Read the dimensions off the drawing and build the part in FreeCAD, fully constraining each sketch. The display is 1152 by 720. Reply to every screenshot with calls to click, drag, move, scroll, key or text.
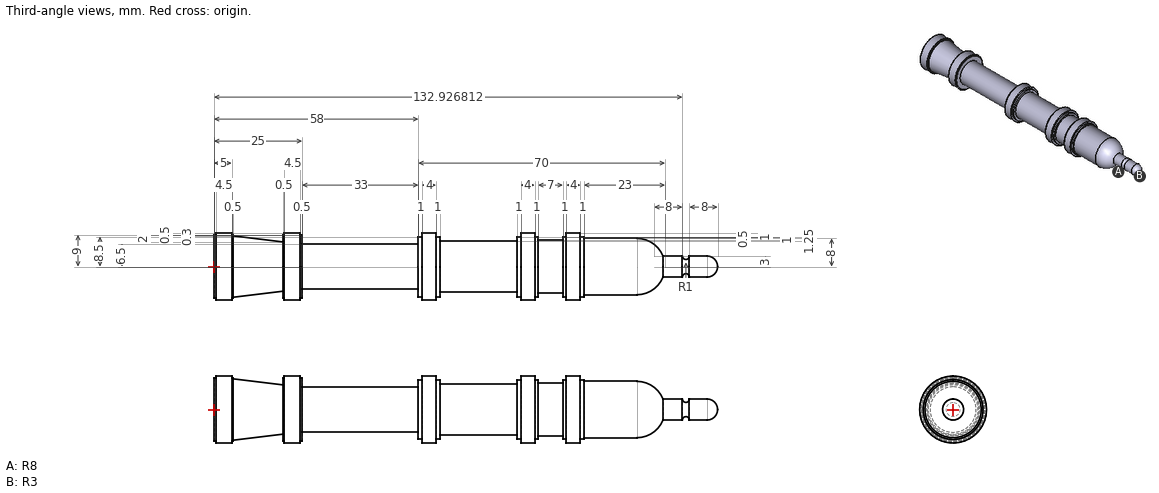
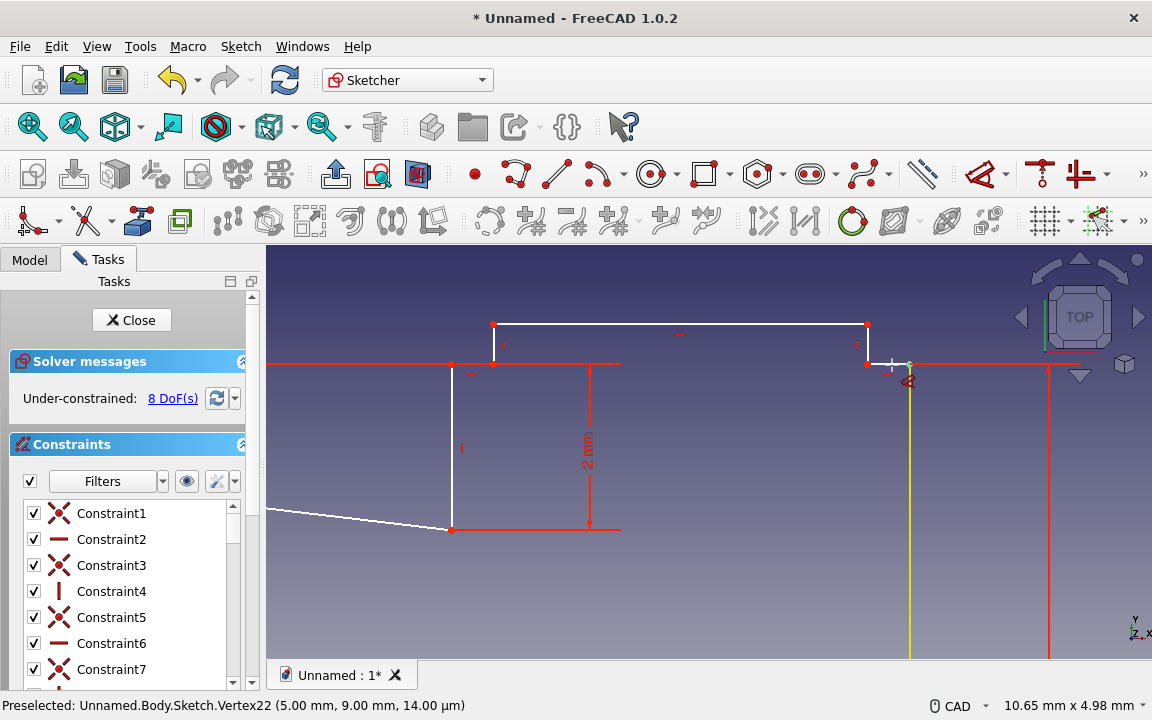
click(889, 364)
click(889, 330)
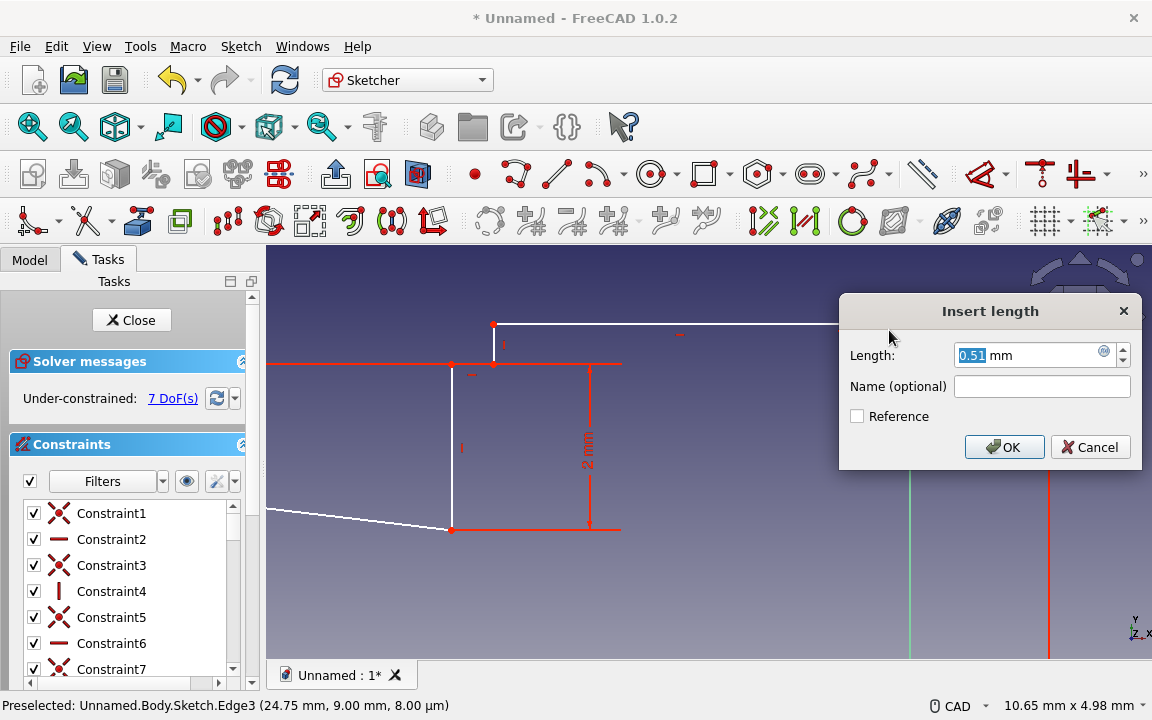
text(0.5)
key(Return)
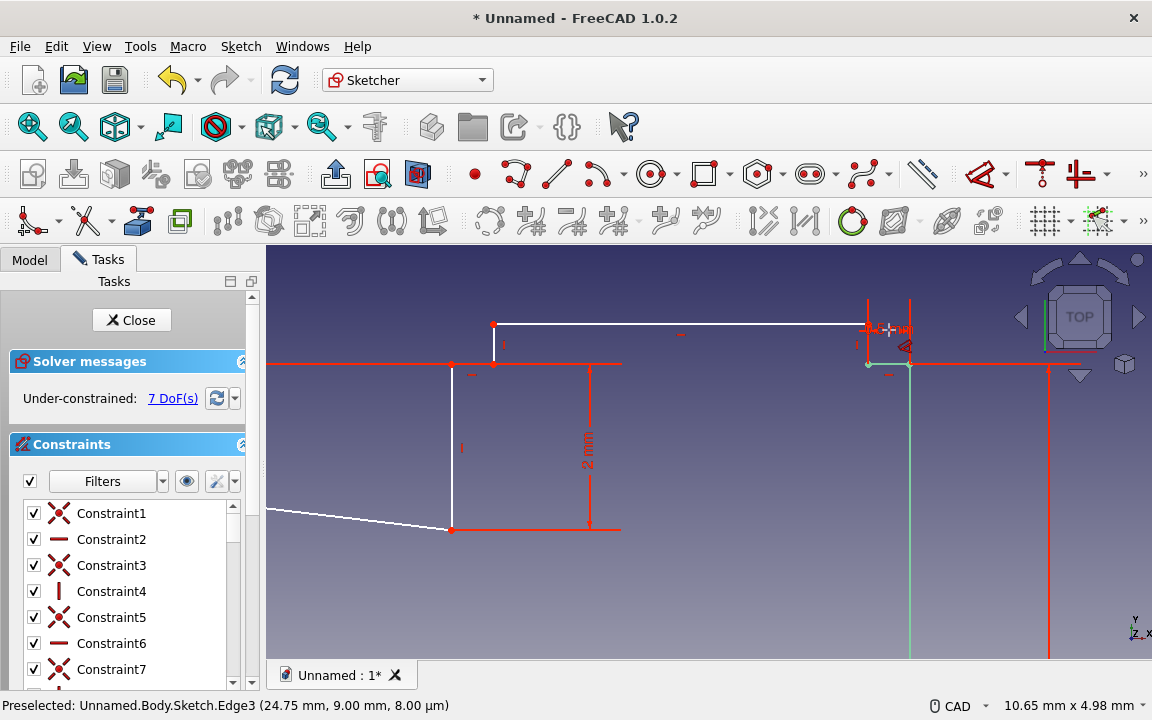
click(868, 352)
click(834, 353)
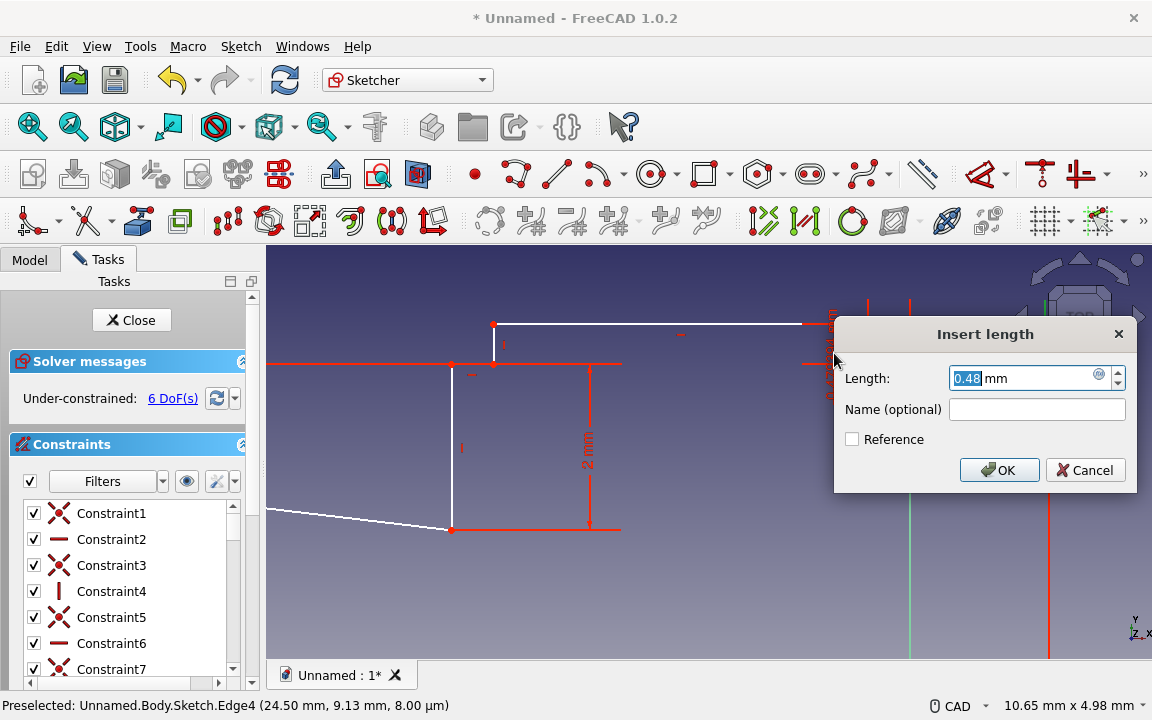
text(0.5)
key(Return)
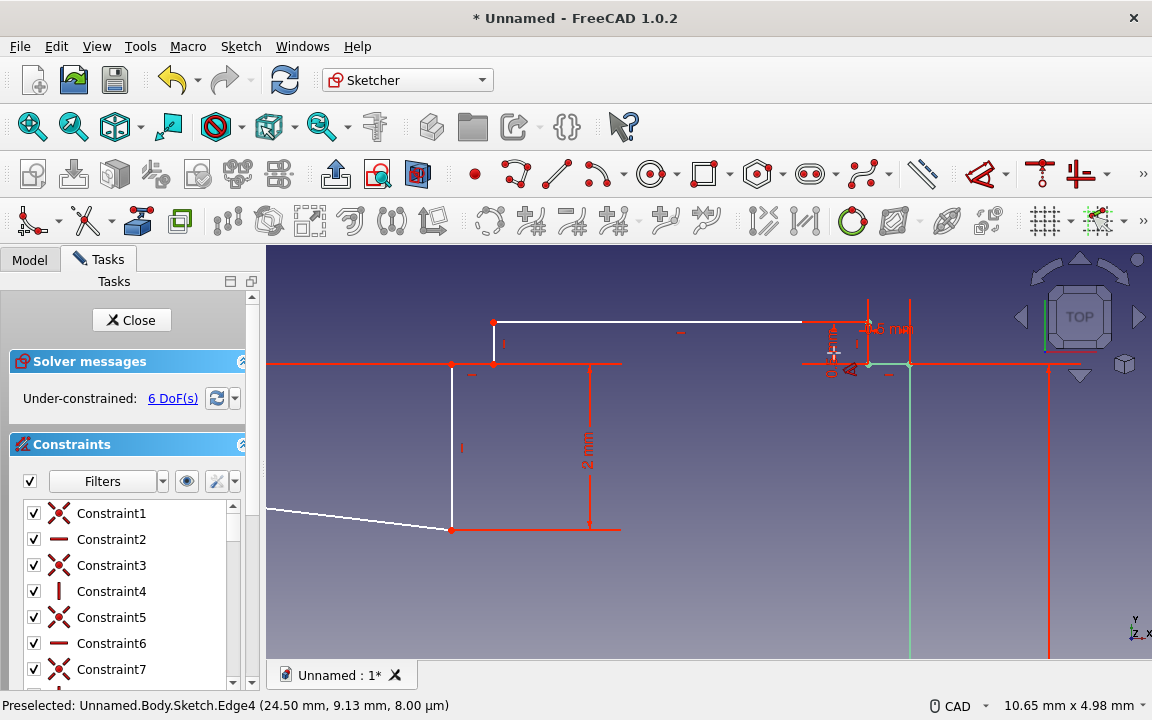
scroll(893, 365, down, 7)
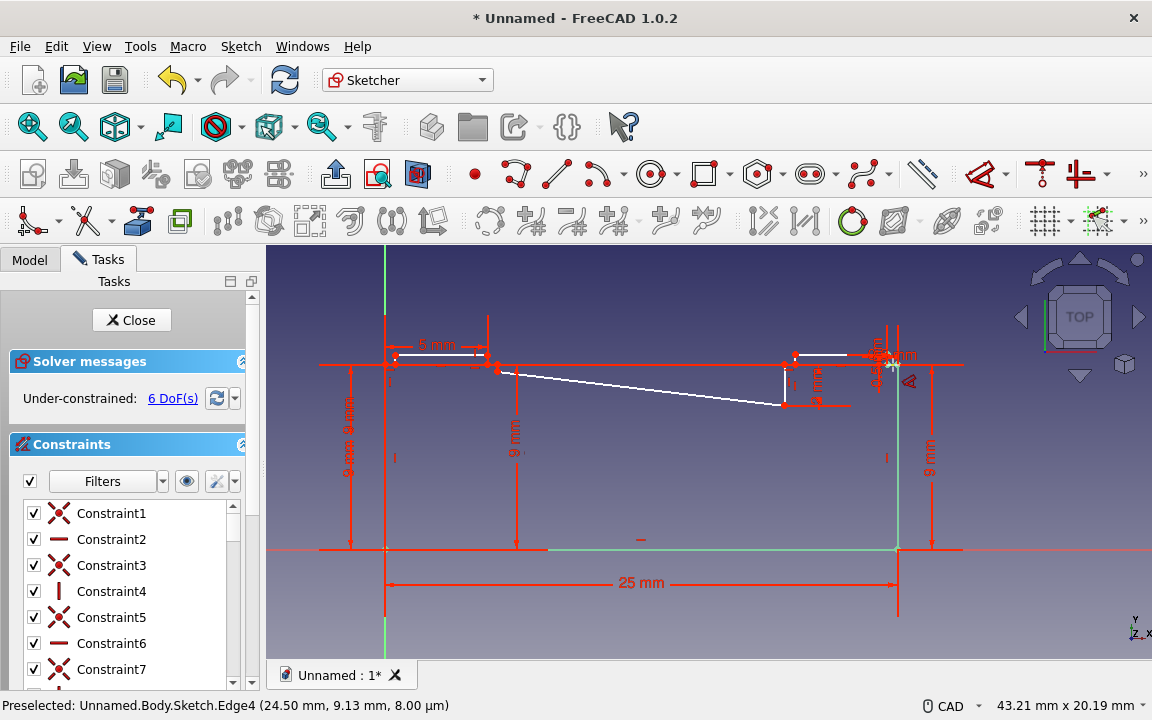
click(860, 355)
click(841, 321)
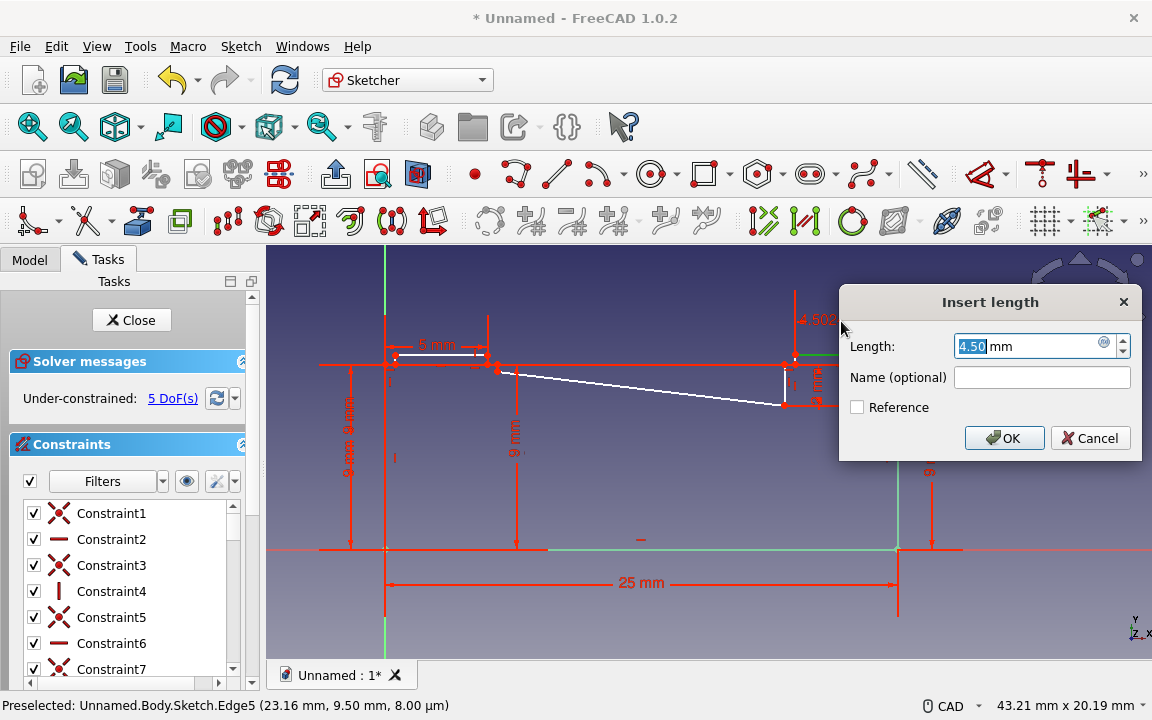
text(4.5)
key(Return)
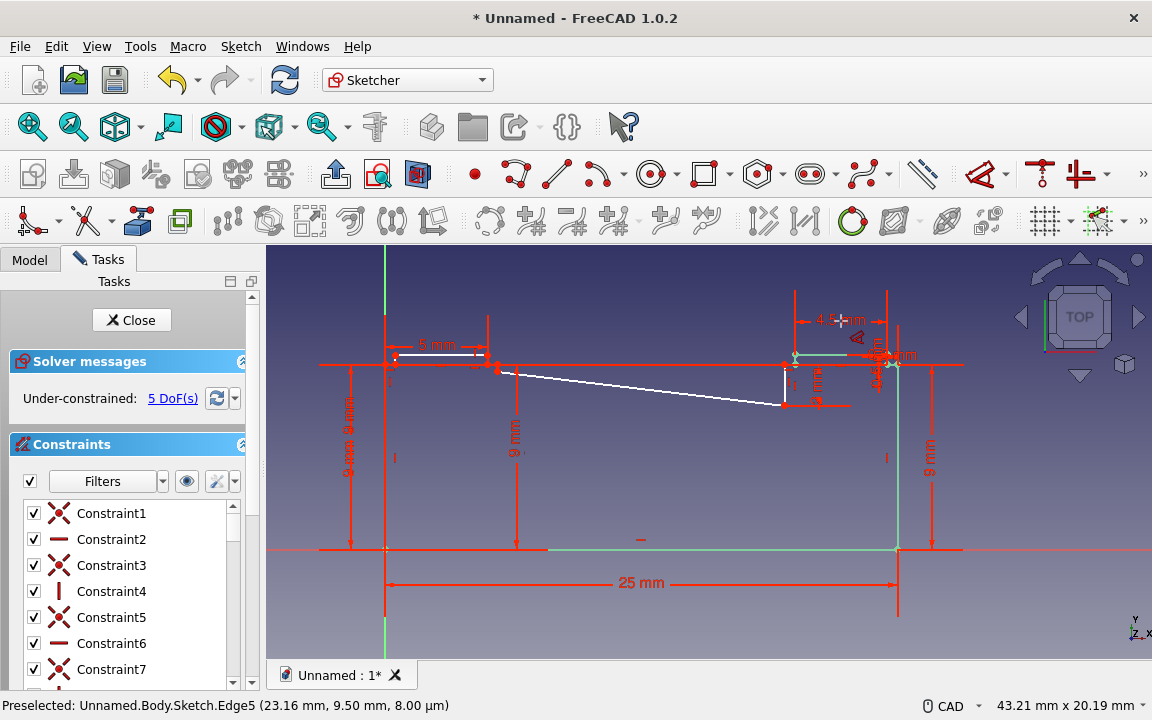
scroll(790, 365, up, 7)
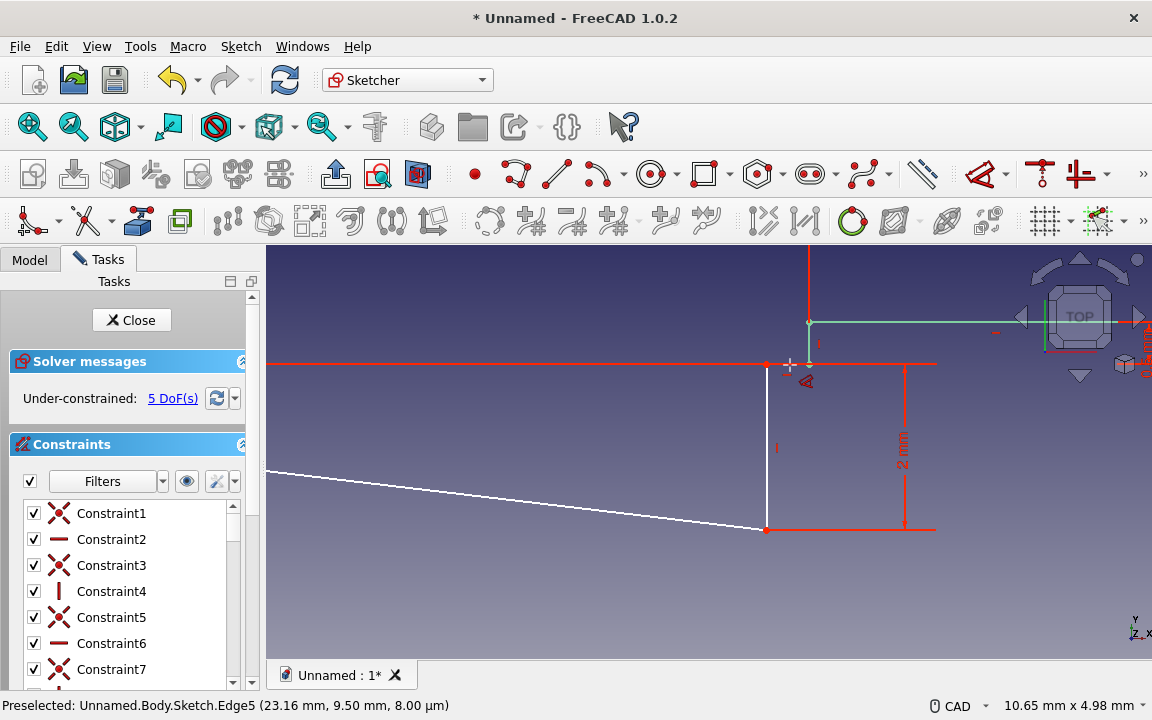
click(788, 364)
click(788, 330)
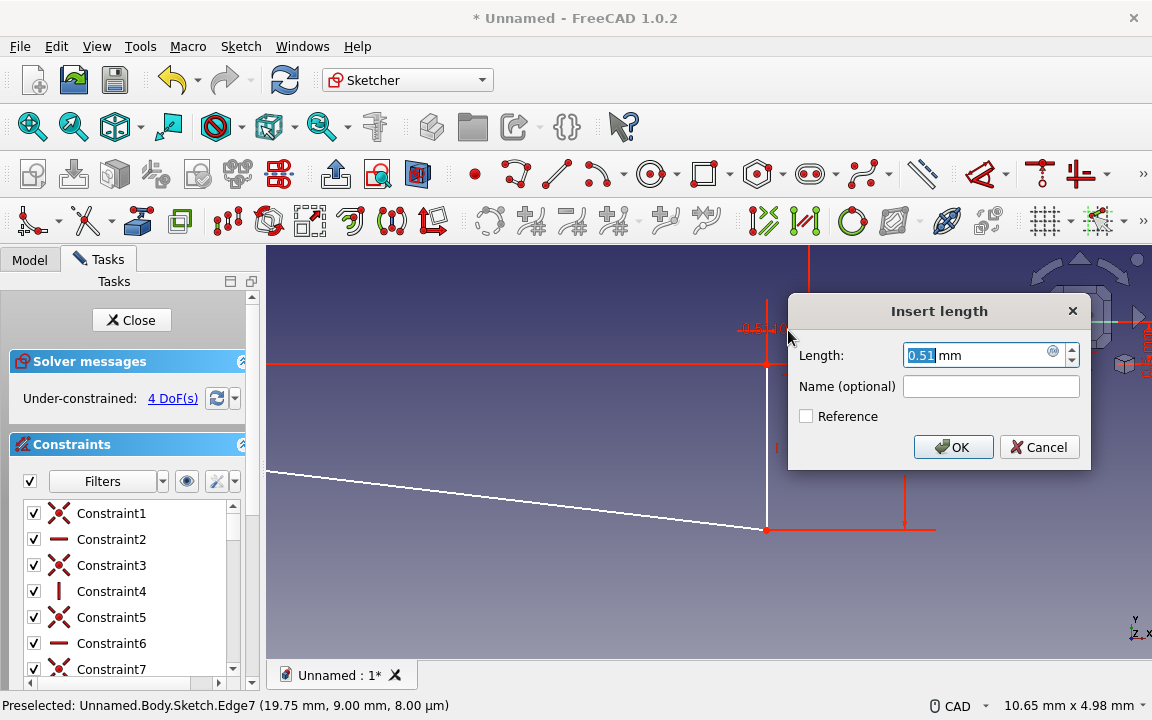
text(0.5)
key(Return)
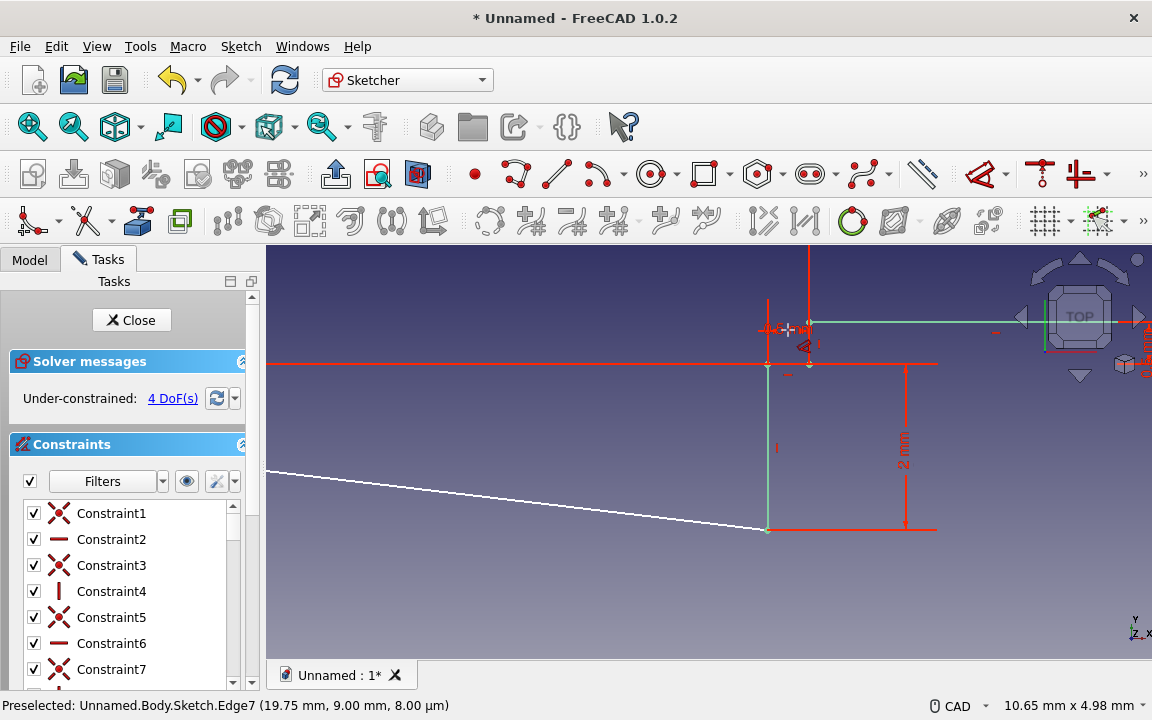
scroll(789, 365, down, 7)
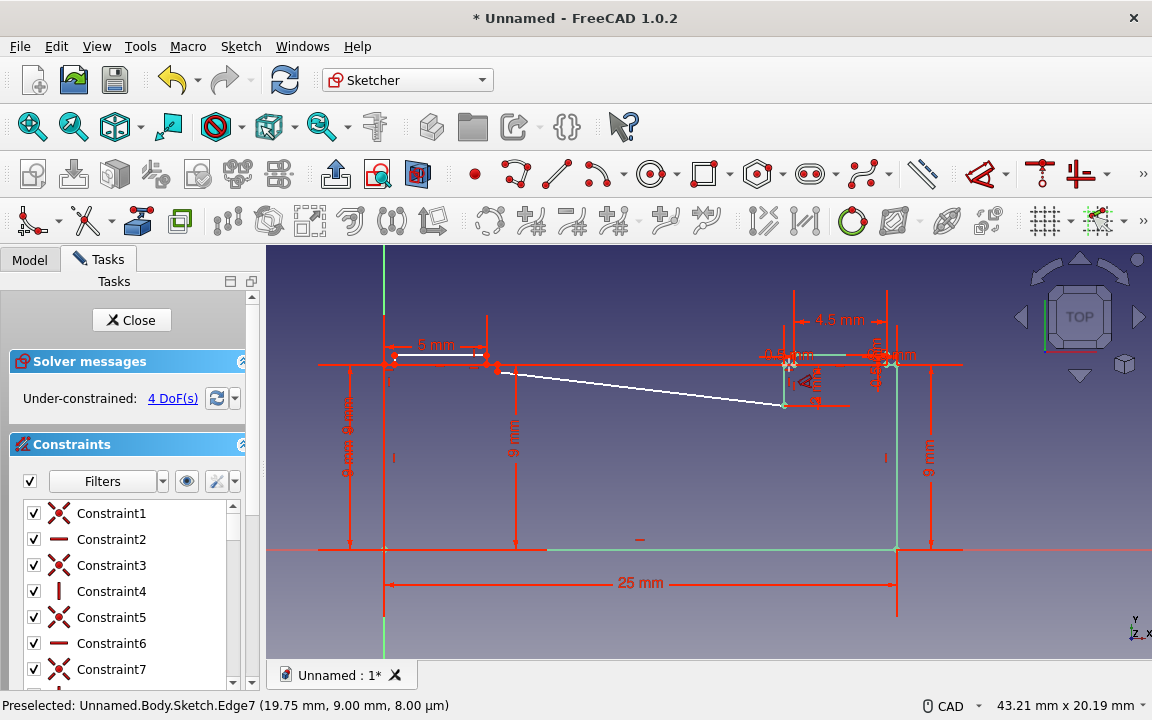
scroll(497, 369, up, 10)